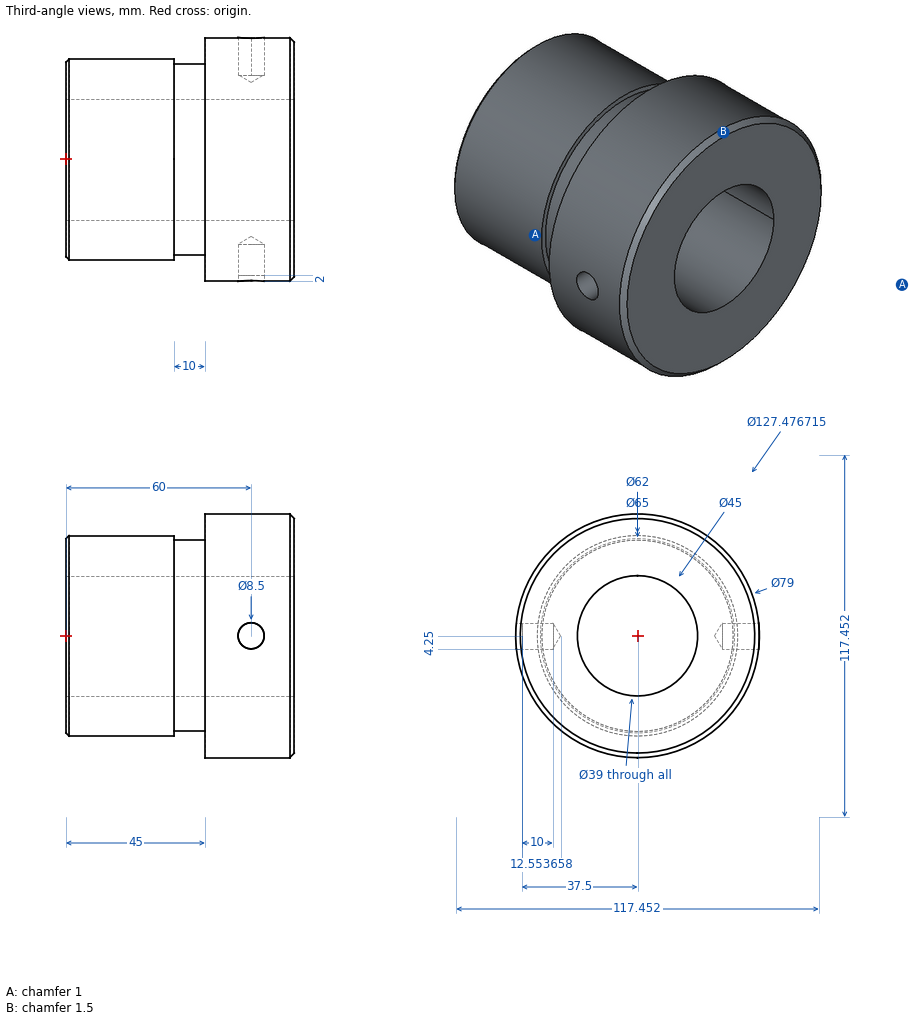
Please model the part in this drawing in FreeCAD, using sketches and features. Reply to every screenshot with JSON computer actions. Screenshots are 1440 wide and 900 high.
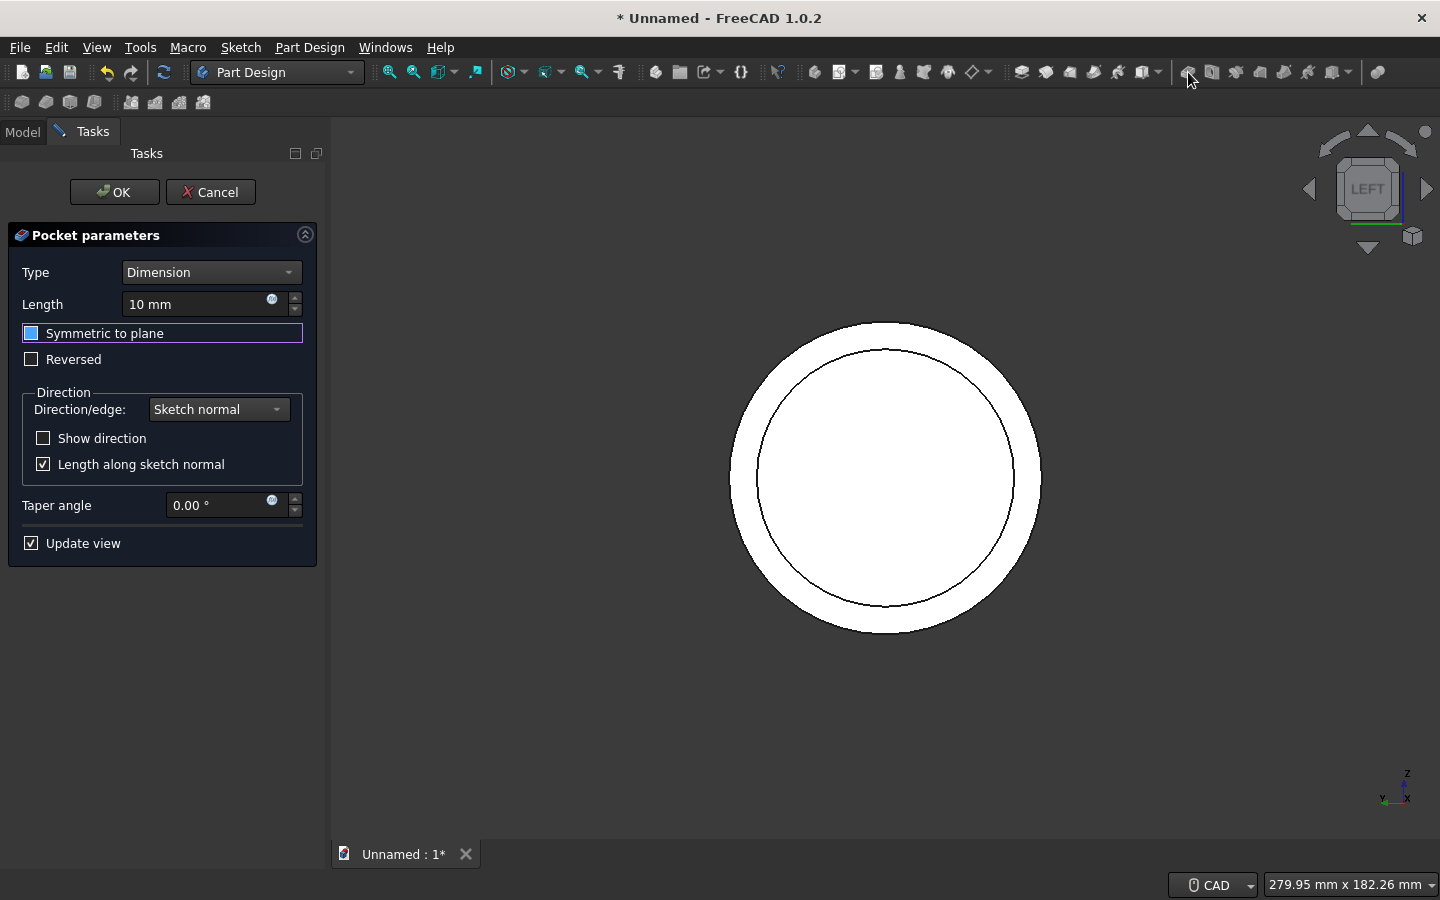
{"action": "left_click", "coordinate": [30, 359]}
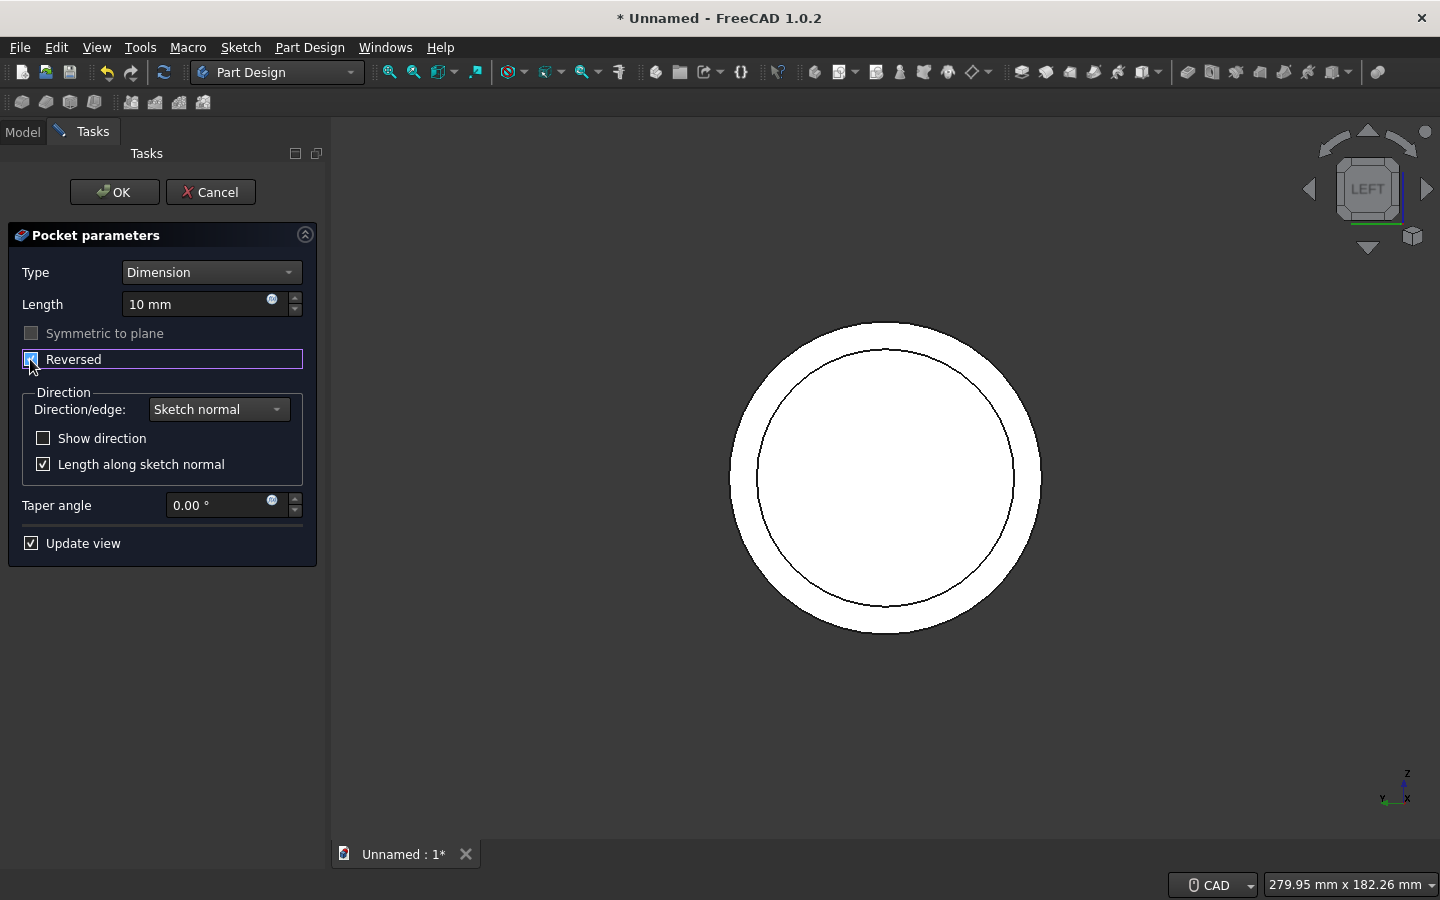
{"action": "left_click", "coordinate": [115, 192]}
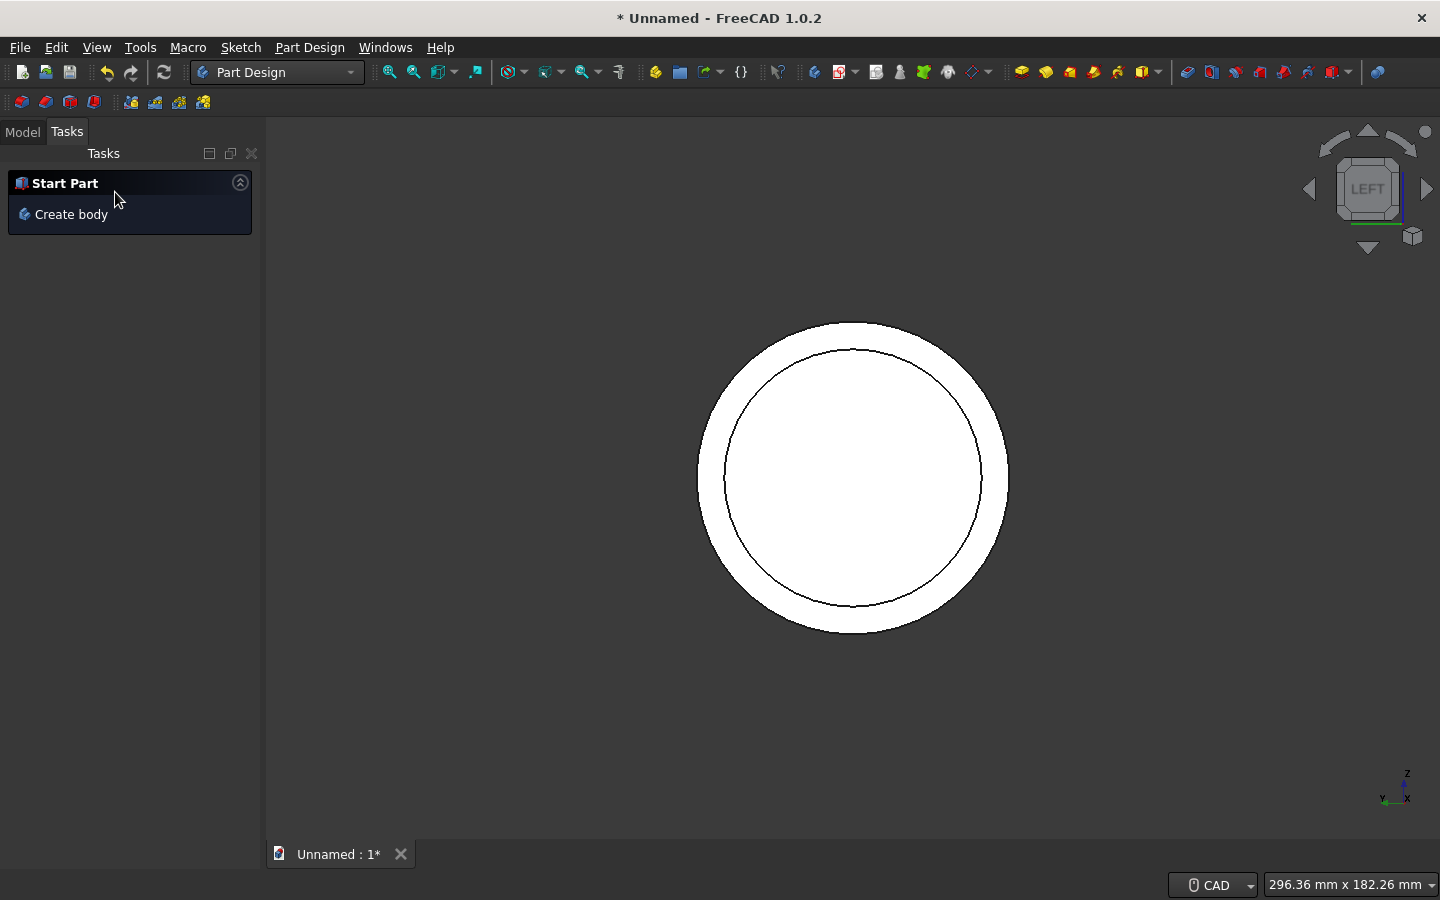
{"action": "key", "text": "v f"}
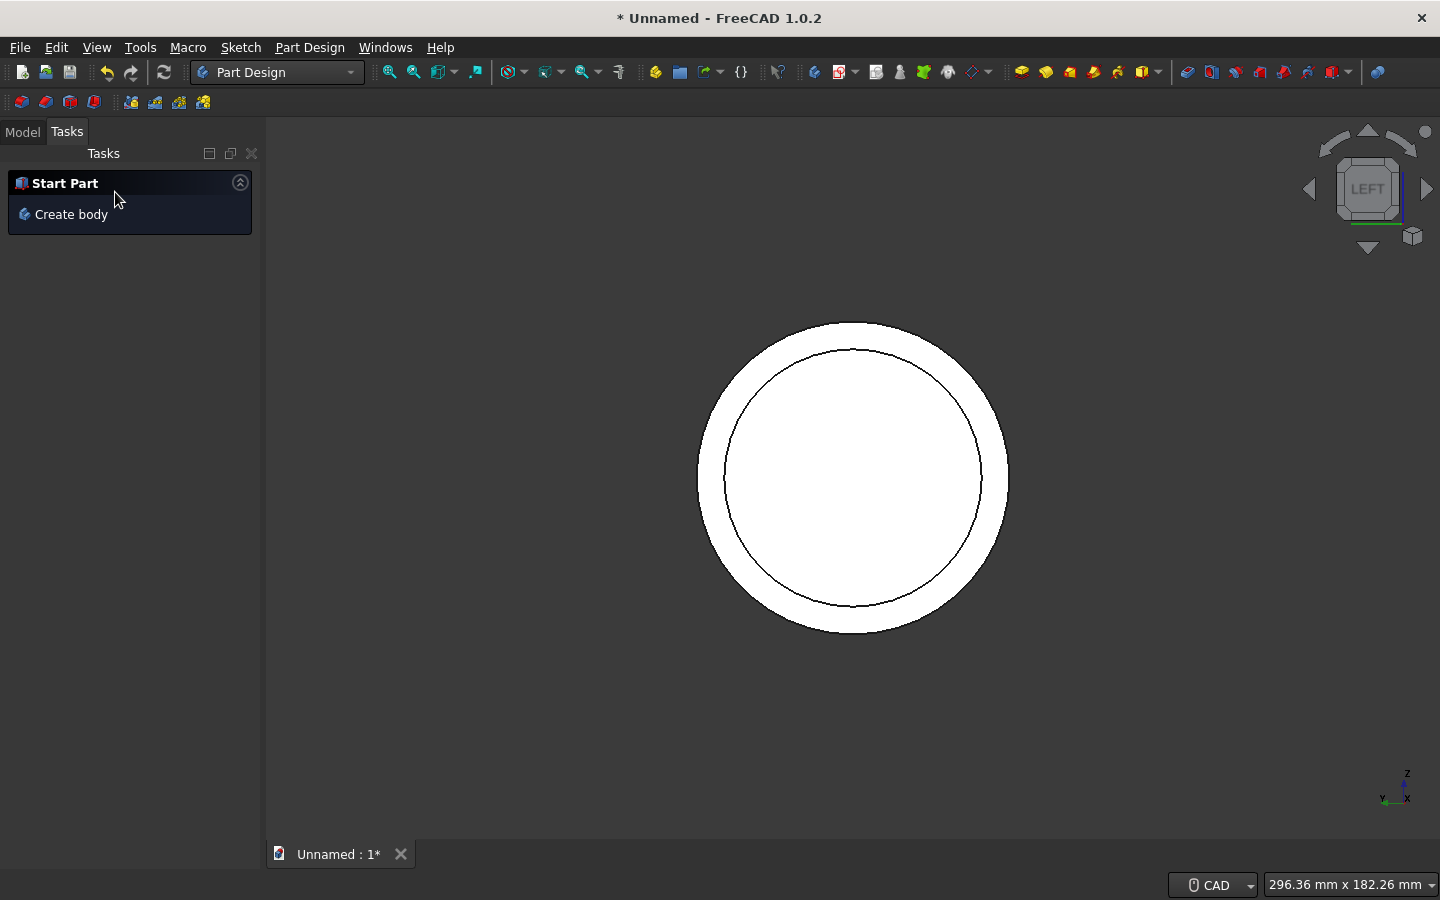
{"action": "left_click", "coordinate": [982, 477]}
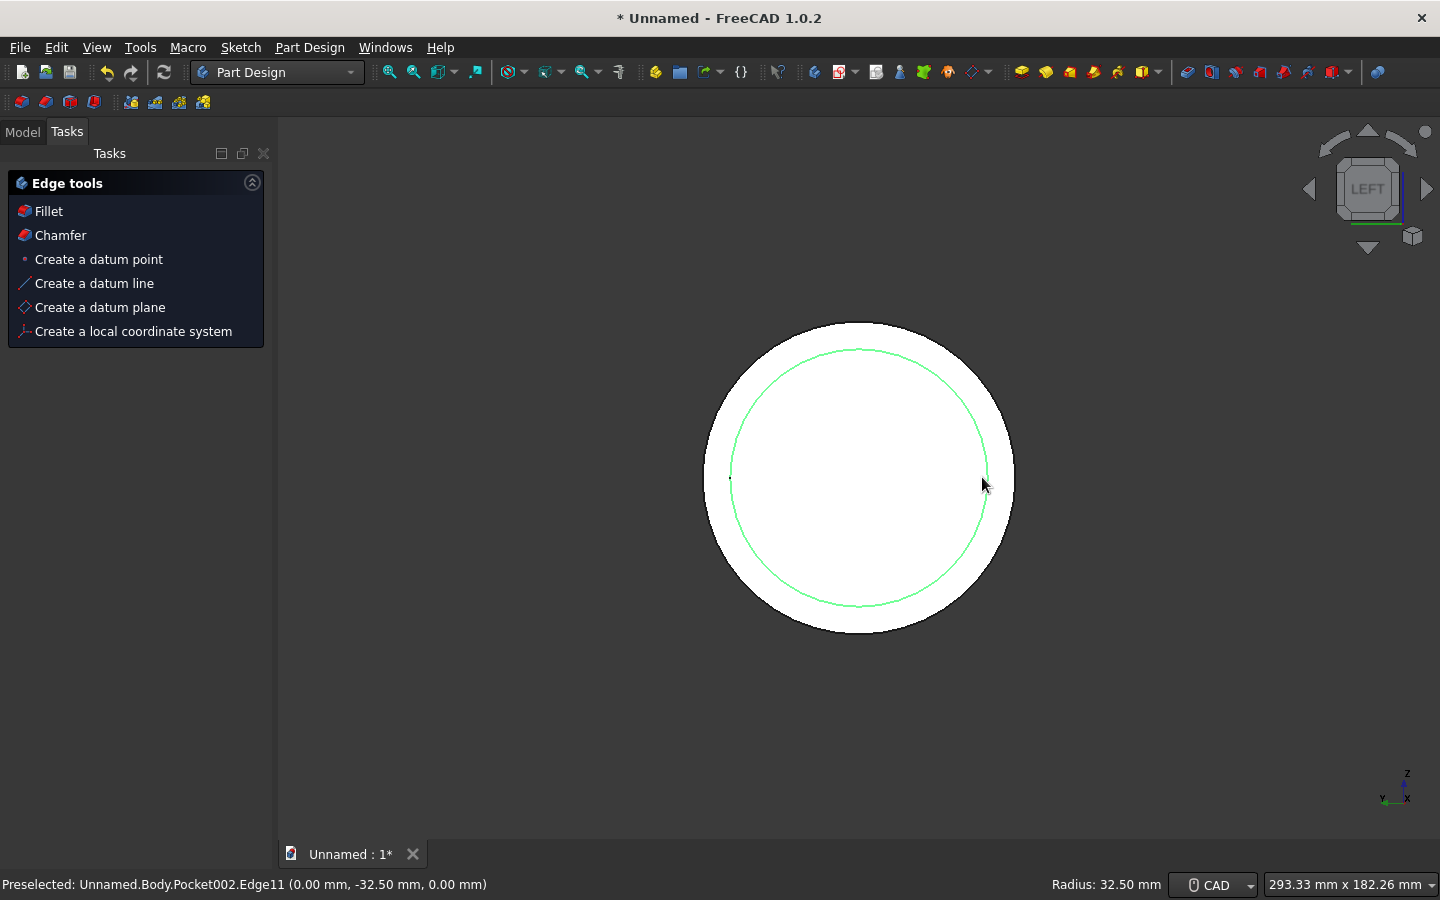
{"action": "key", "text": "0"}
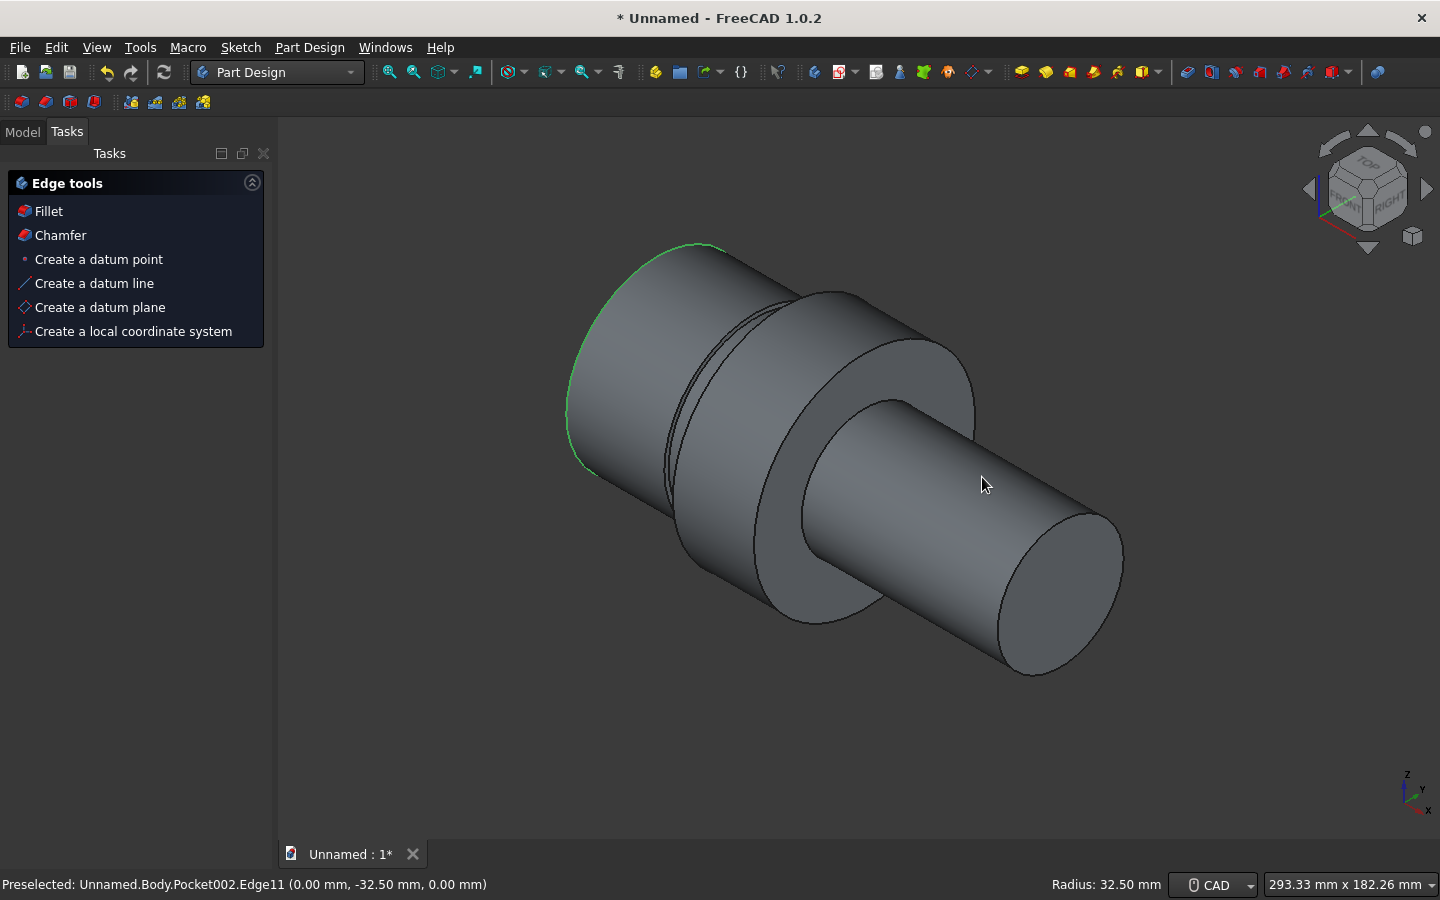
{"action": "left_click", "coordinate": [998, 630], "text": "ctrl"}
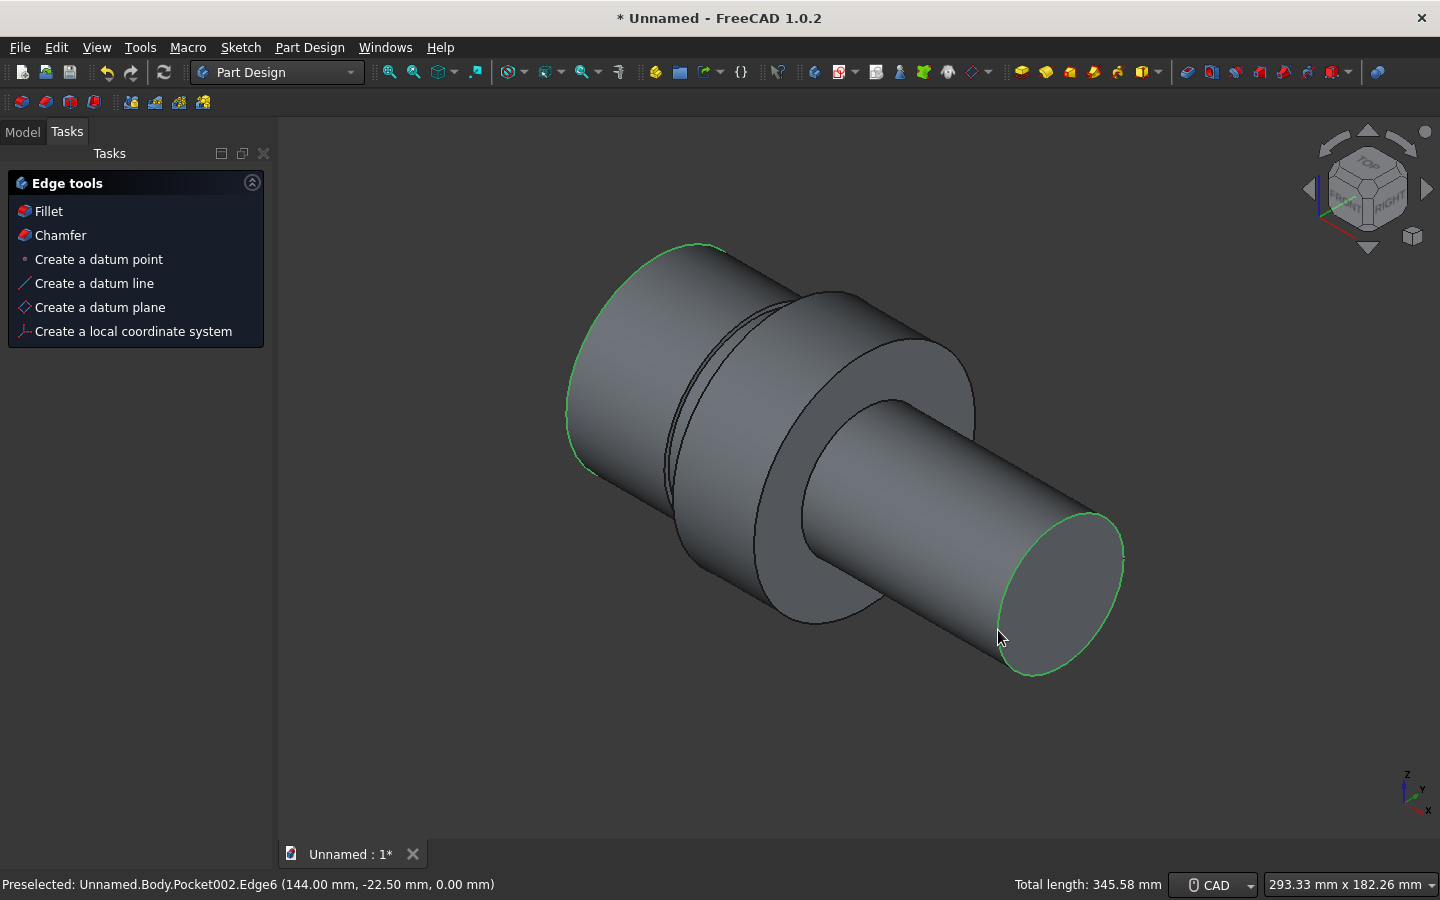
{"action": "left_click", "coordinate": [46, 102]}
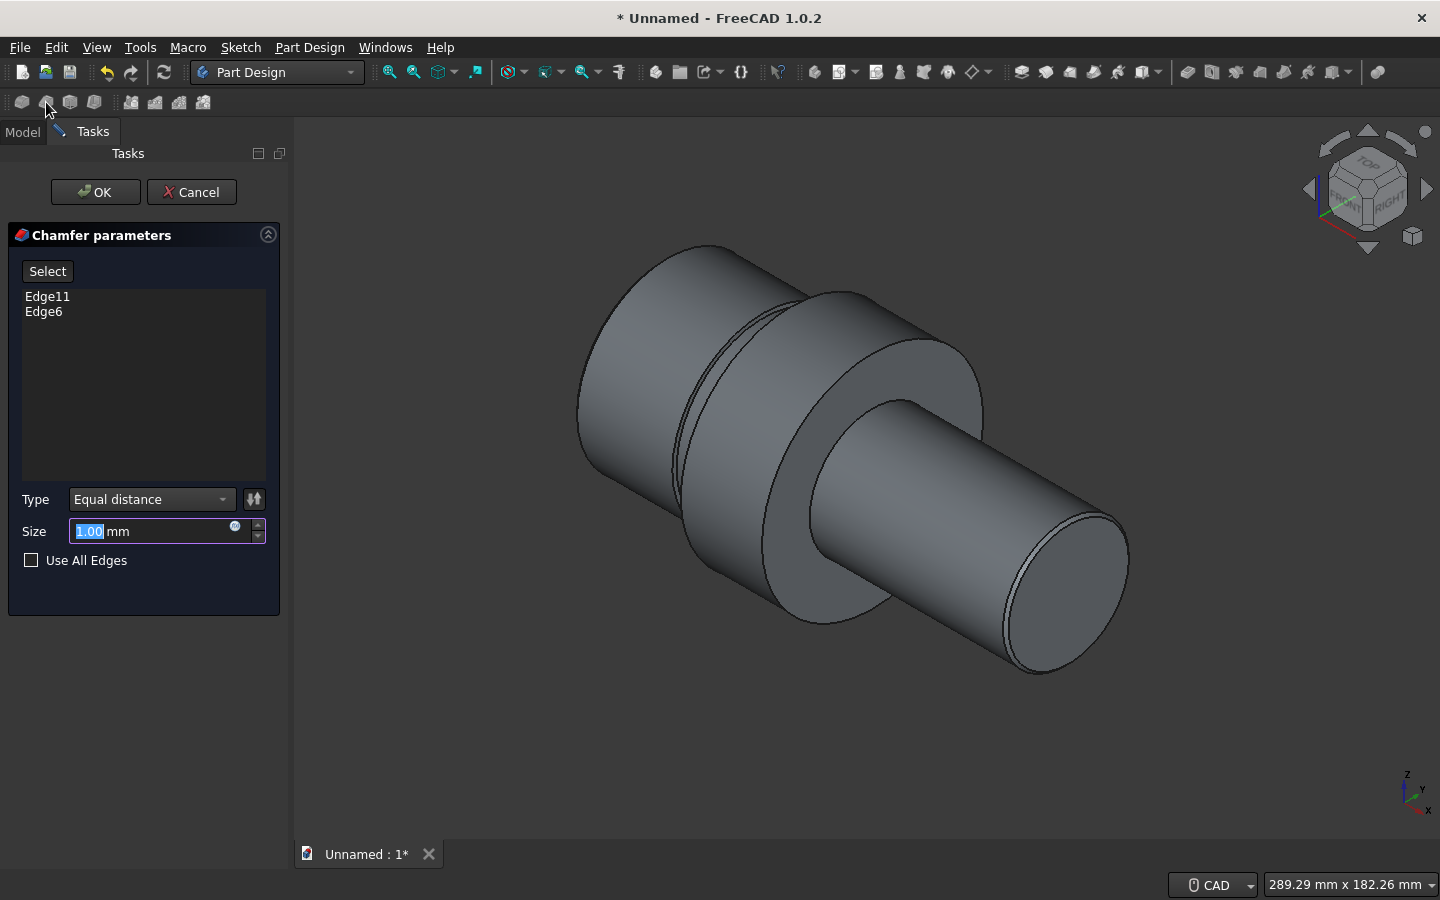
{"action": "type", "text": "1"}
{"action": "key", "text": "Tab"}